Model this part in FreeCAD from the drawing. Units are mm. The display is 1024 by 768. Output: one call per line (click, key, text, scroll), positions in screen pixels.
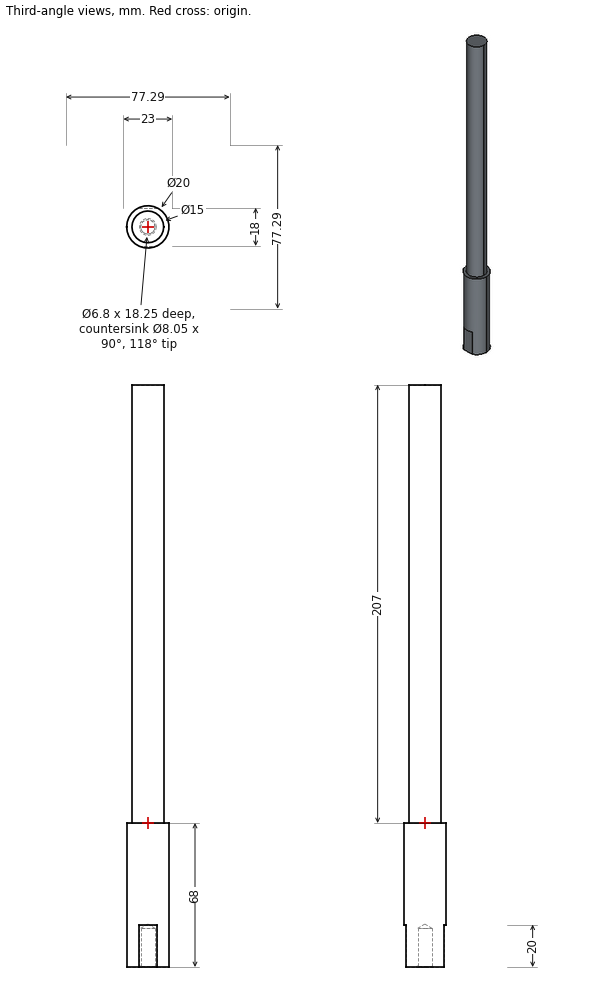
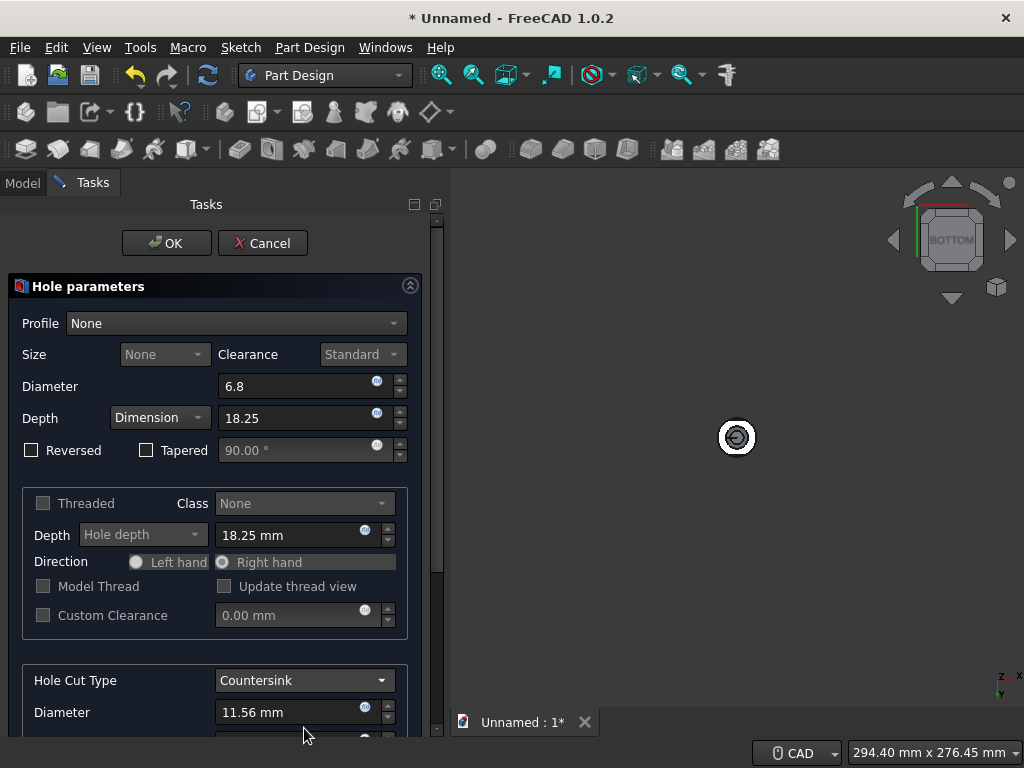
triple_click(298, 712)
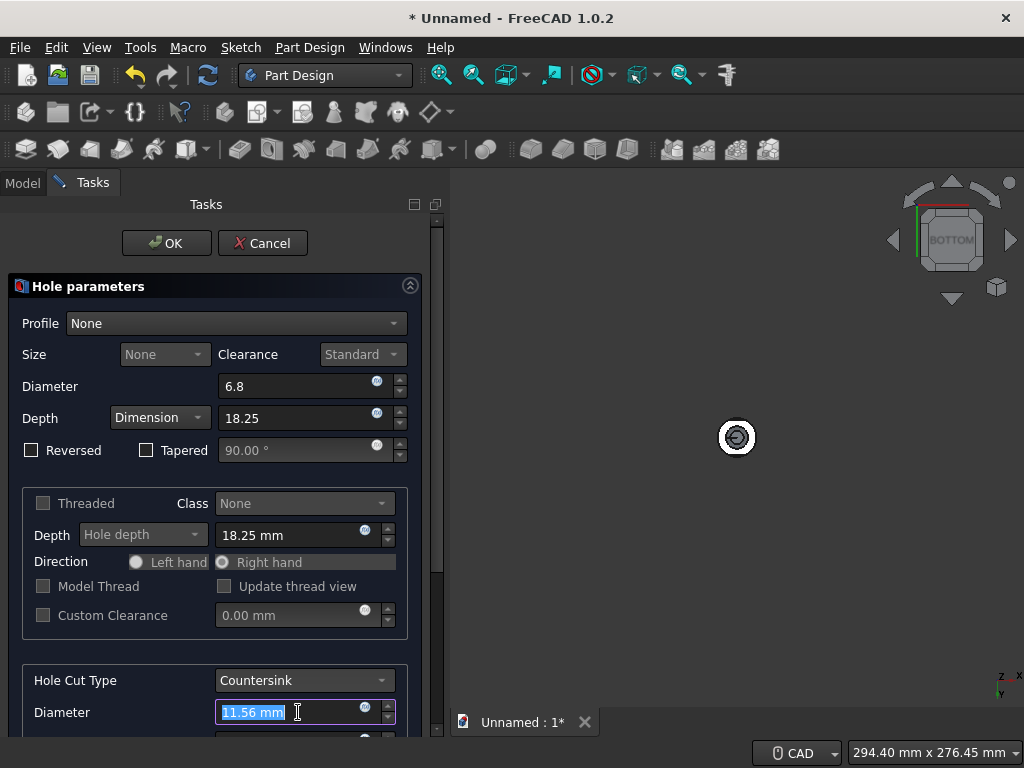
text(8.05)
key(Tab)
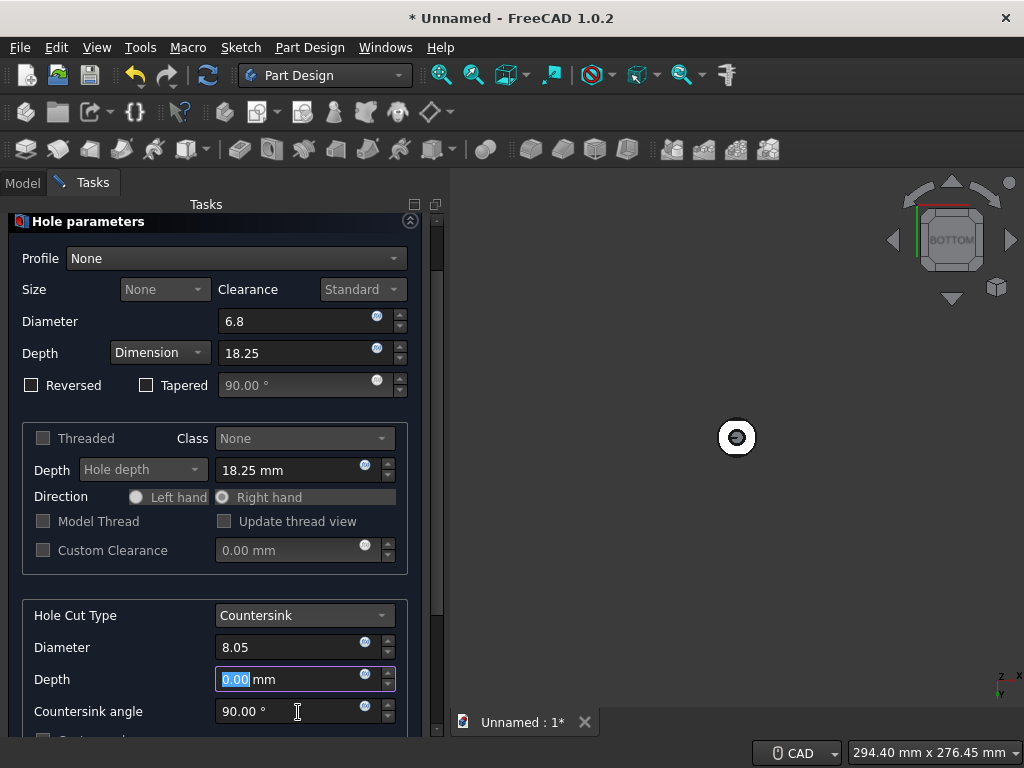
scroll(437, 475, up, 2)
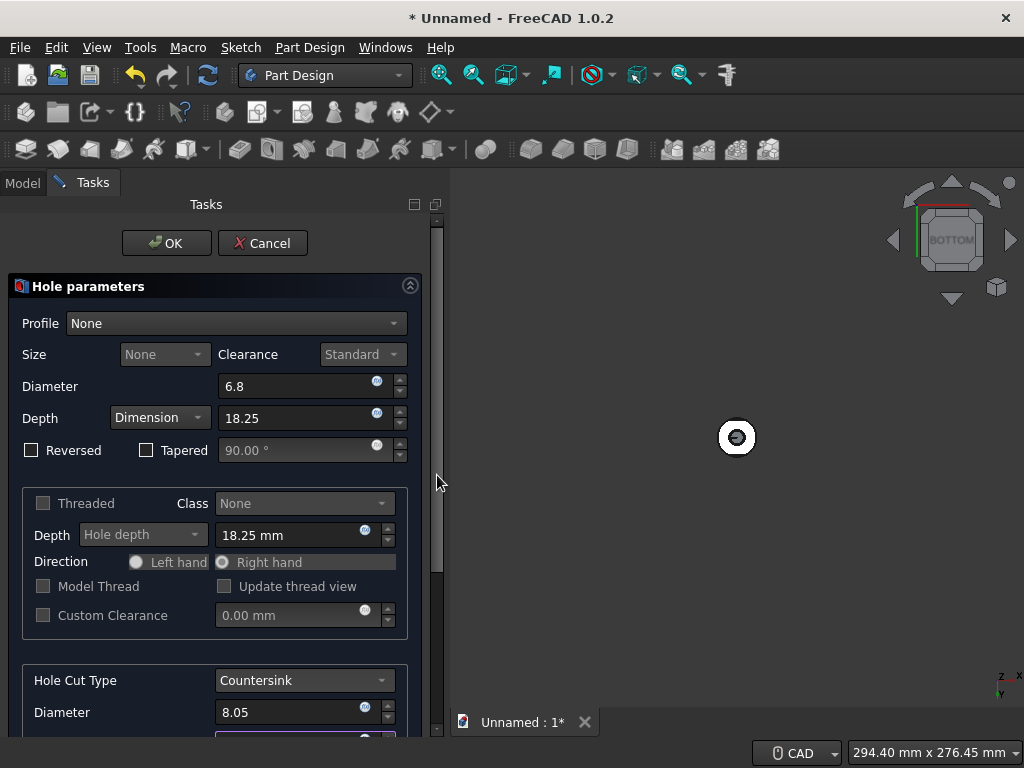
click(167, 243)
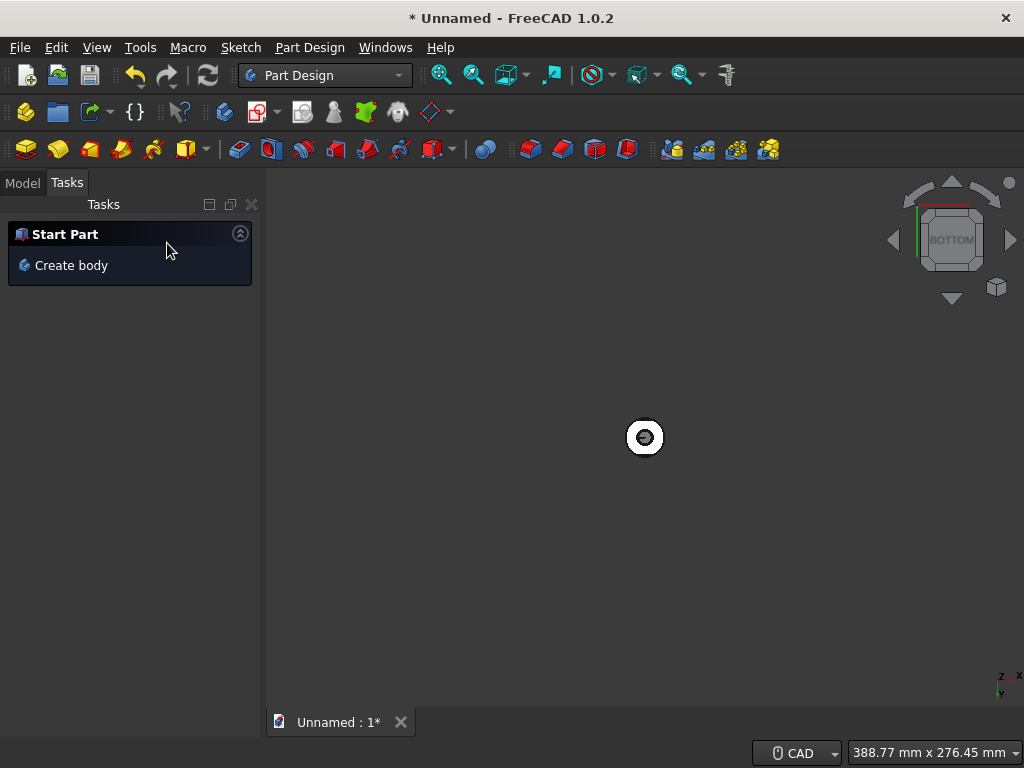
key(0)